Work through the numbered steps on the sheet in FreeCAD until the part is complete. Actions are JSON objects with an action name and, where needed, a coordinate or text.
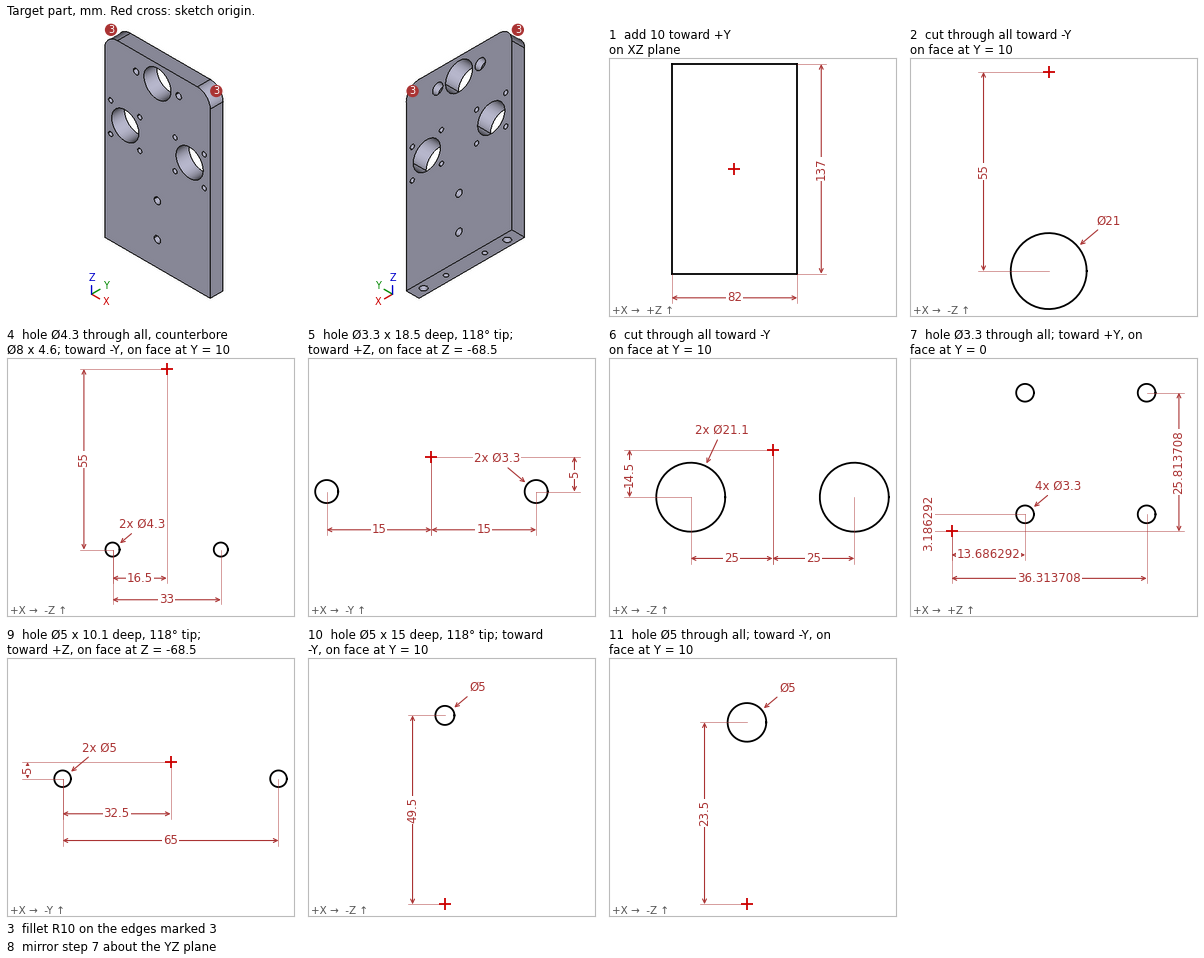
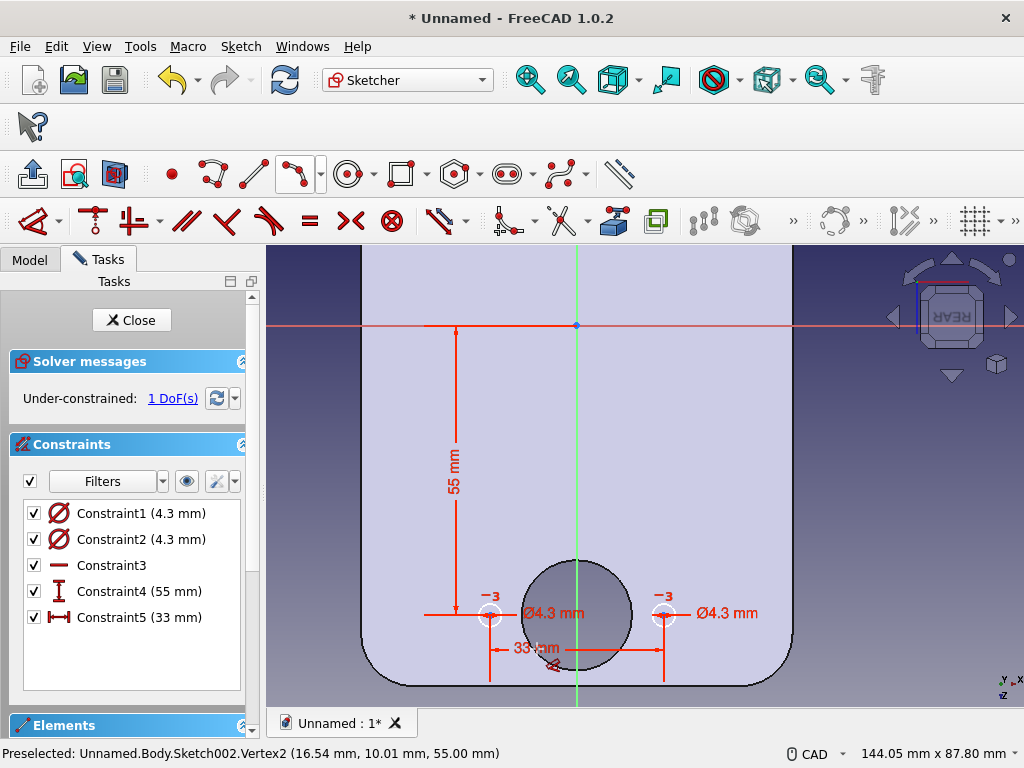
{"action": "left_click", "coordinate": [490, 615]}
{"action": "left_click", "coordinate": [534, 292]}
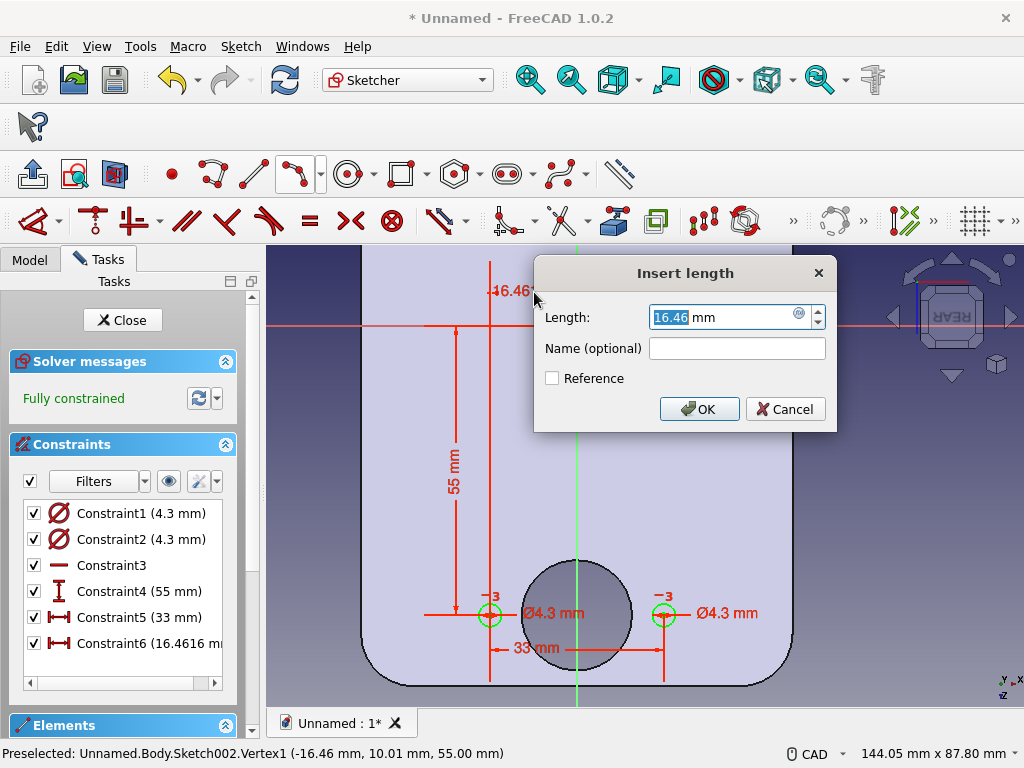
{"action": "type", "text": "16.5"}
{"action": "key", "text": "Return"}
{"action": "key", "text": "Escape"}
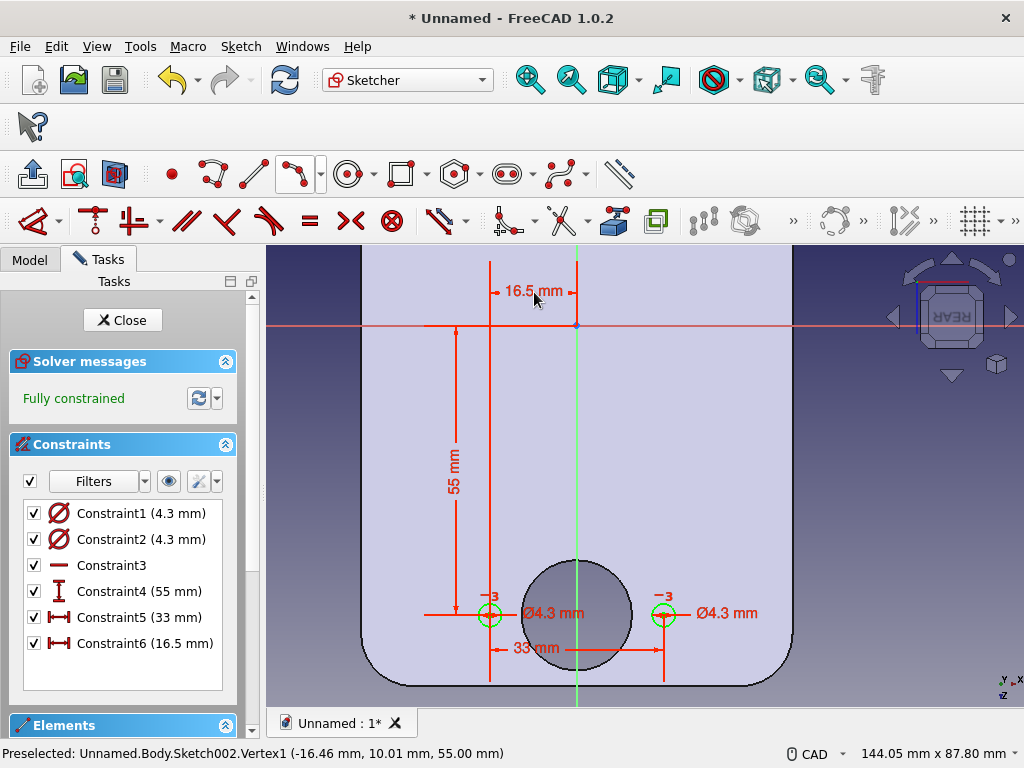
{"action": "left_click", "coordinate": [123, 320]}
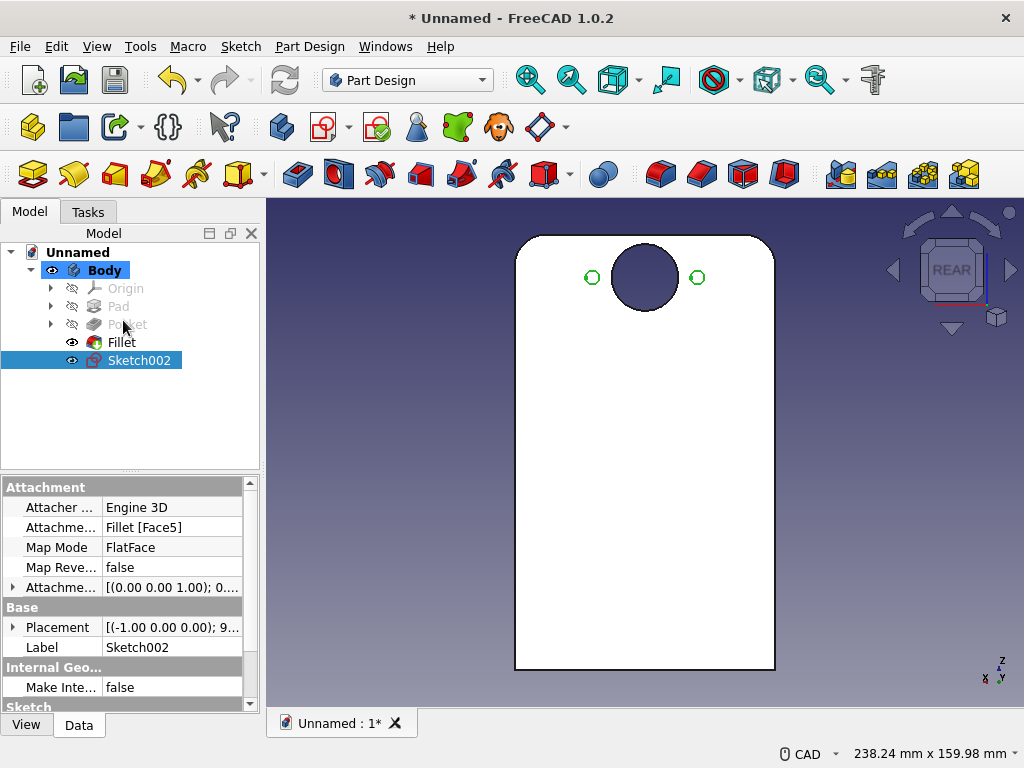
{"action": "left_click", "coordinate": [339, 174]}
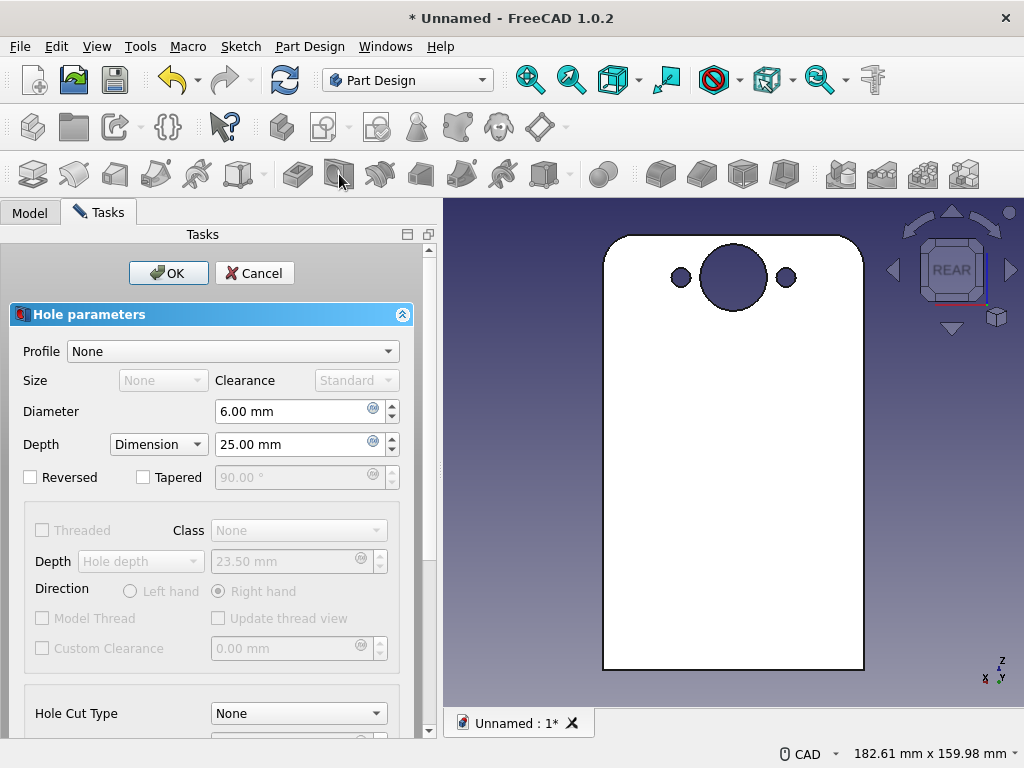
{"action": "triple_click", "coordinate": [300, 412]}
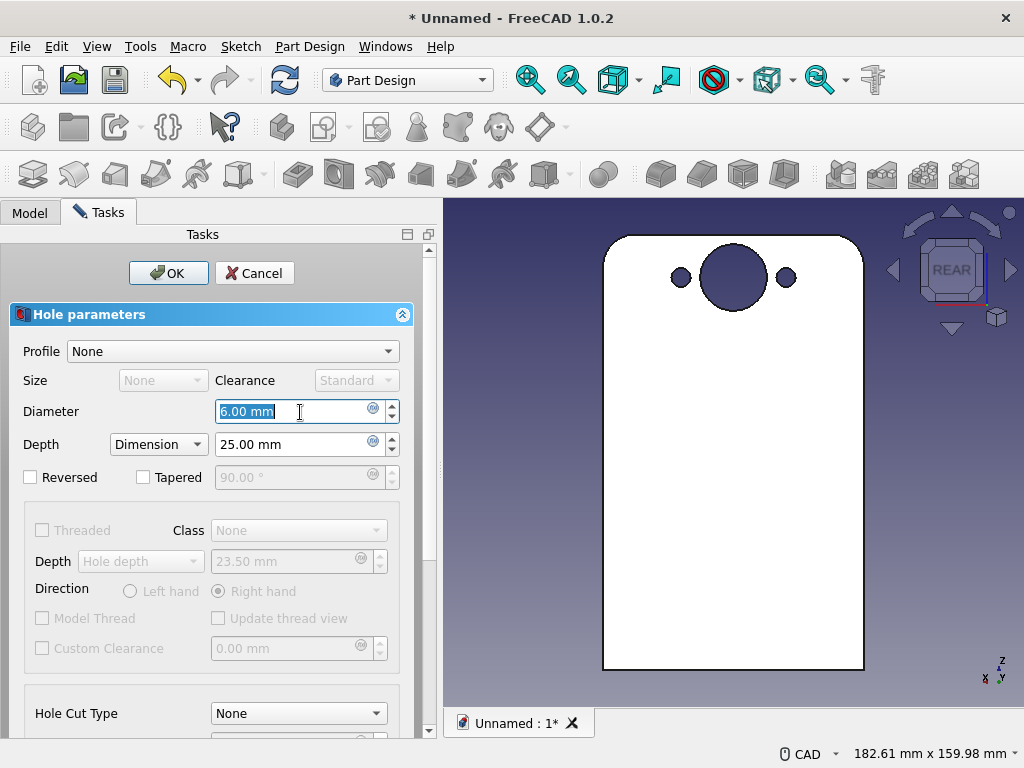
{"action": "type", "text": "4.3"}
{"action": "key", "text": "Tab"}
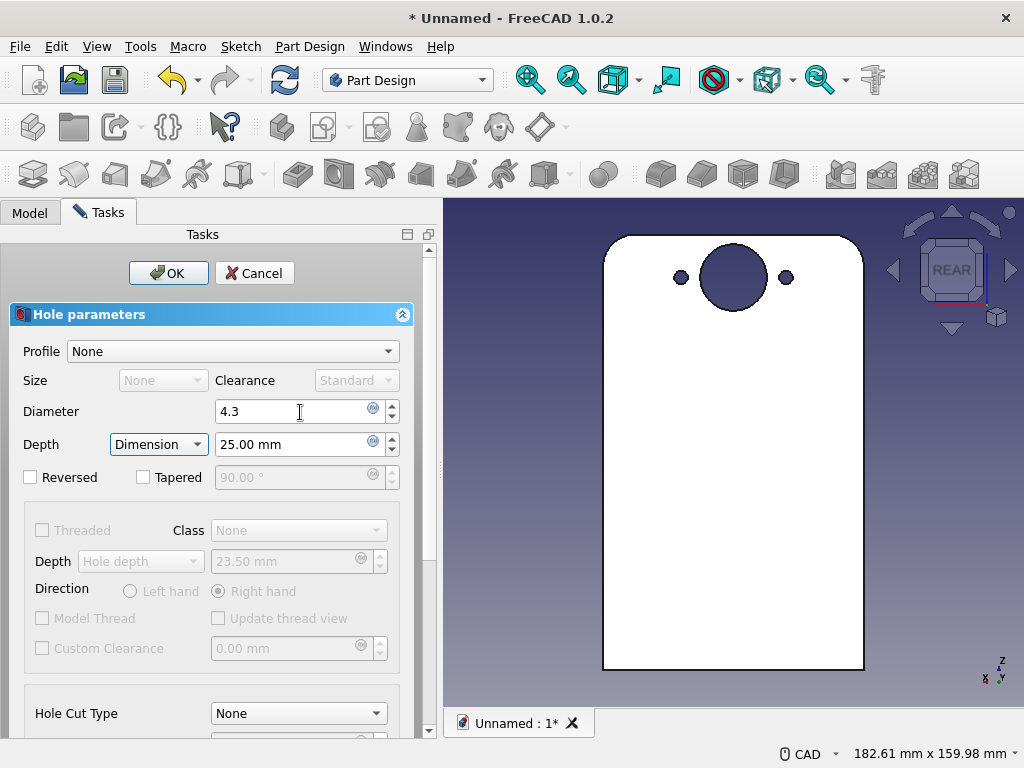
{"action": "left_click", "coordinate": [160, 444]}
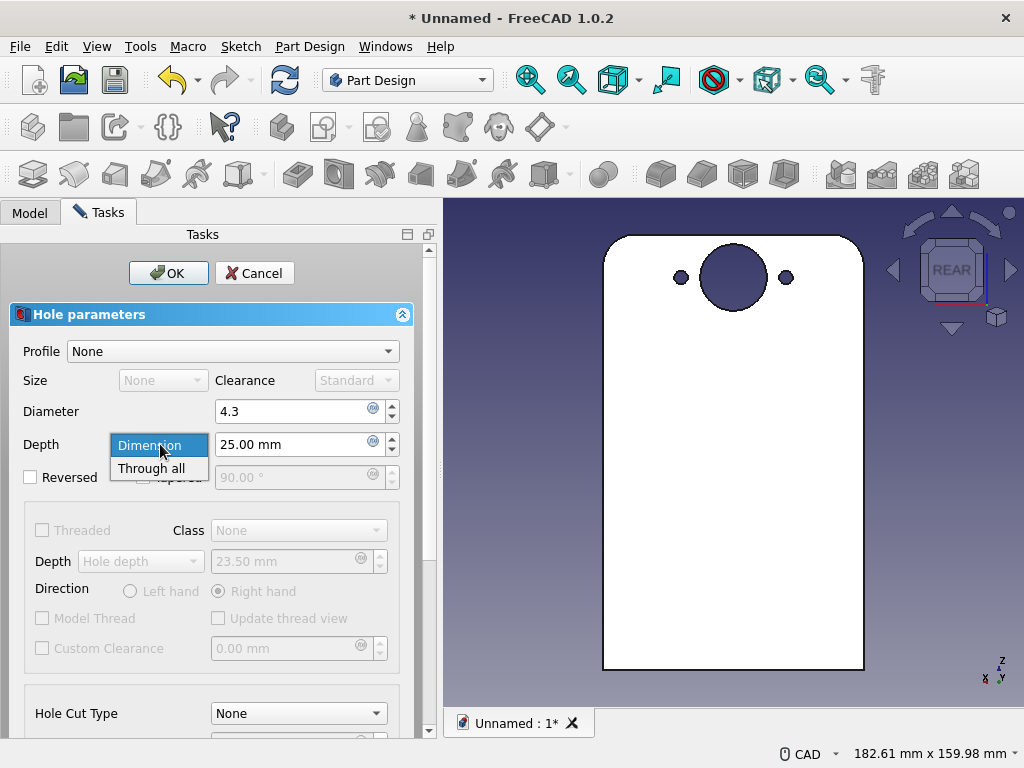
{"action": "left_click", "coordinate": [158, 468]}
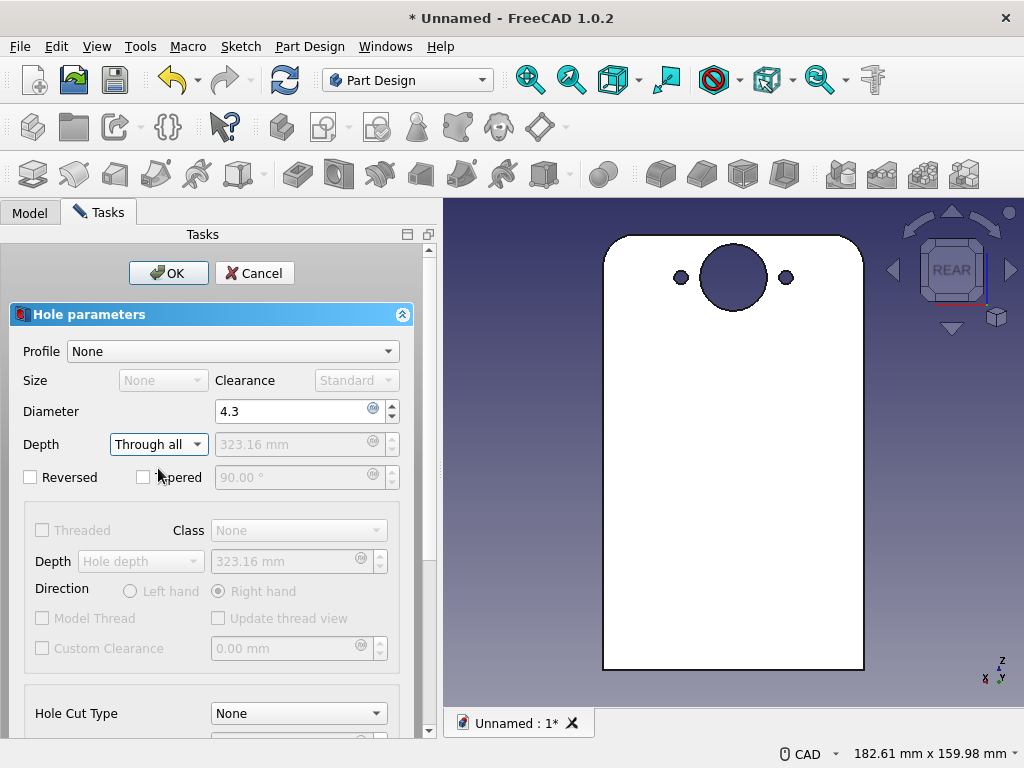
{"action": "left_click", "coordinate": [300, 714]}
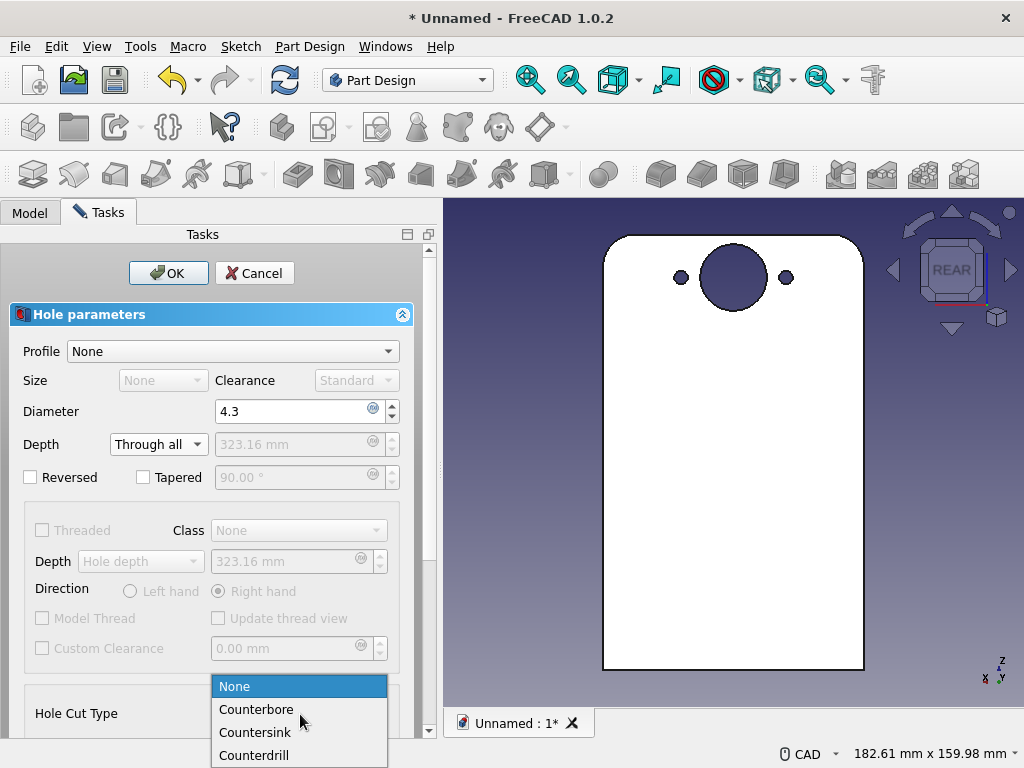
{"action": "left_click", "coordinate": [298, 710]}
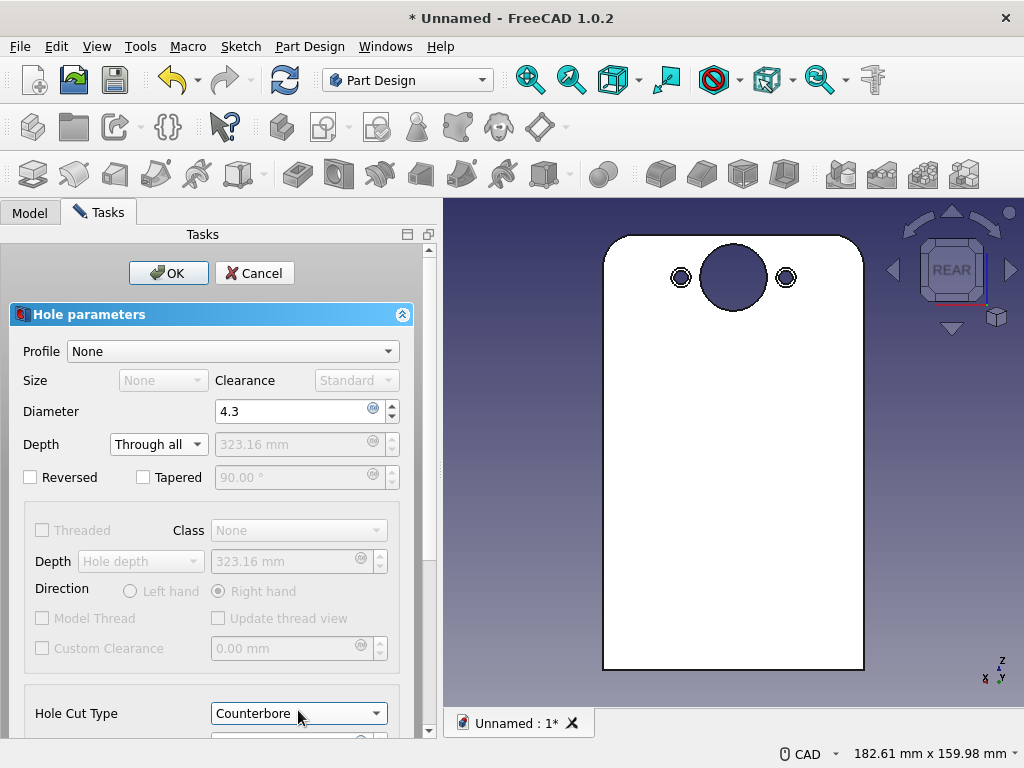
{"action": "scroll", "coordinate": [429, 491], "scroll_direction": "down", "scroll_amount": 2}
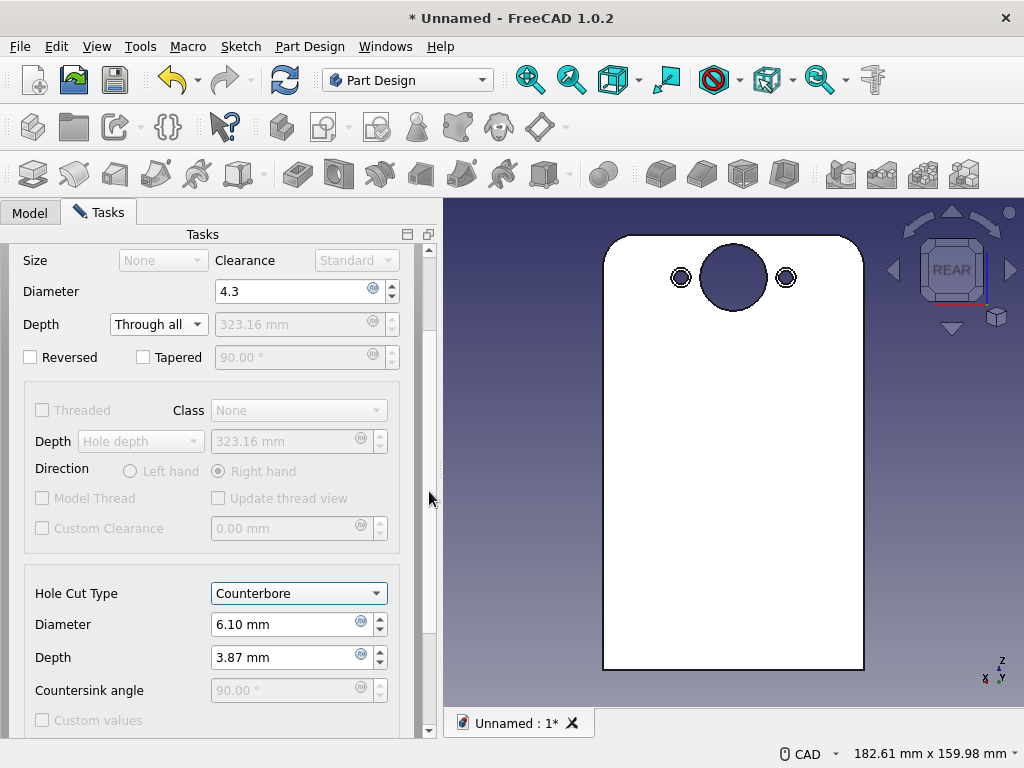
{"action": "triple_click", "coordinate": [292, 624]}